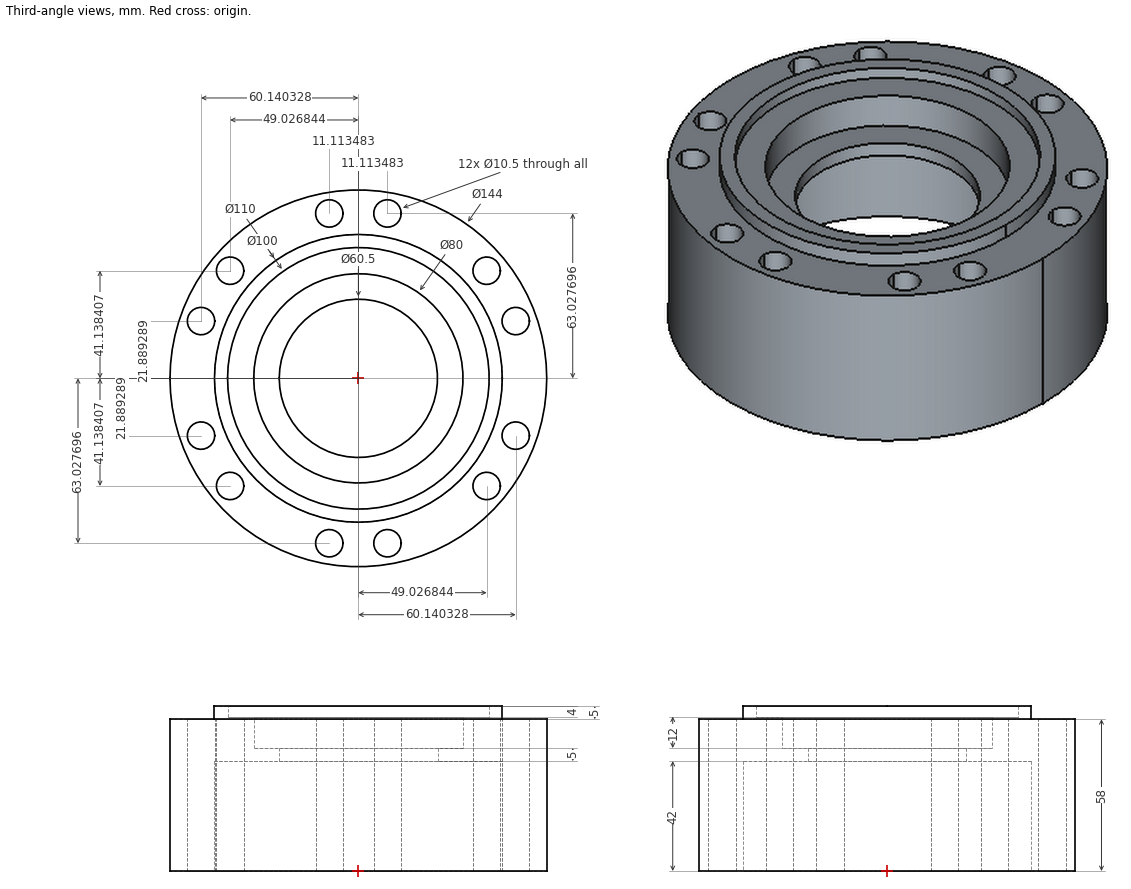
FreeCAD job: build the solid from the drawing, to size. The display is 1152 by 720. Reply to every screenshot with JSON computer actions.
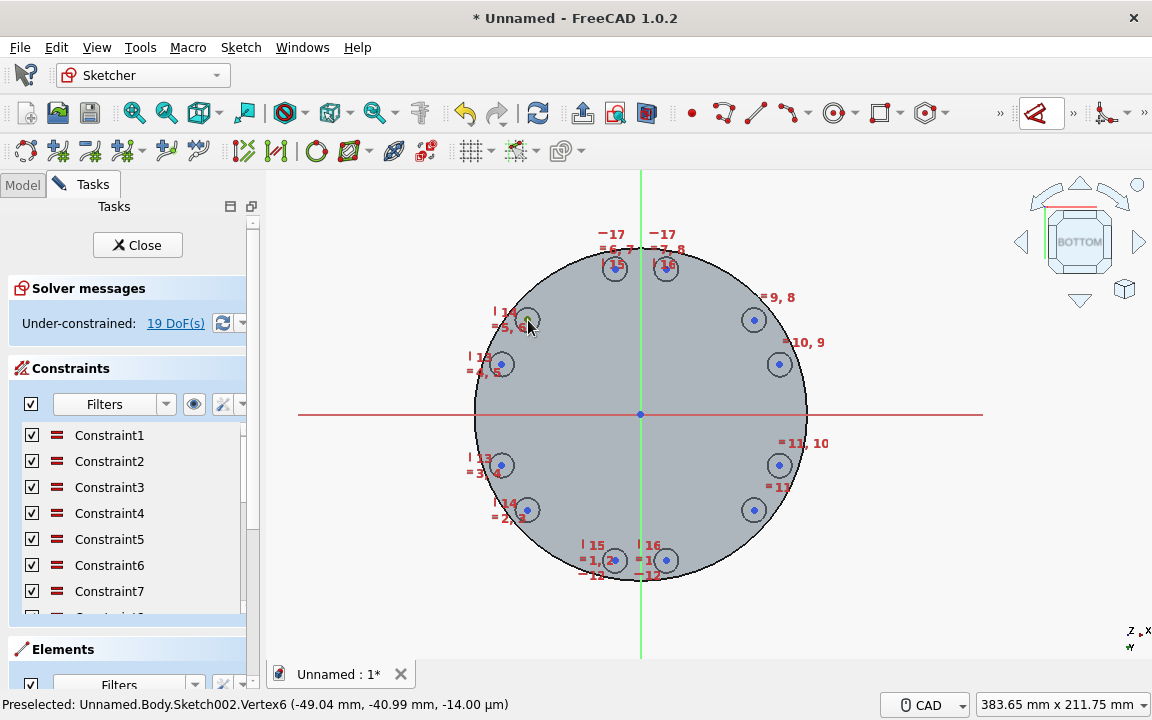
{"action": "left_click", "coordinate": [754, 320]}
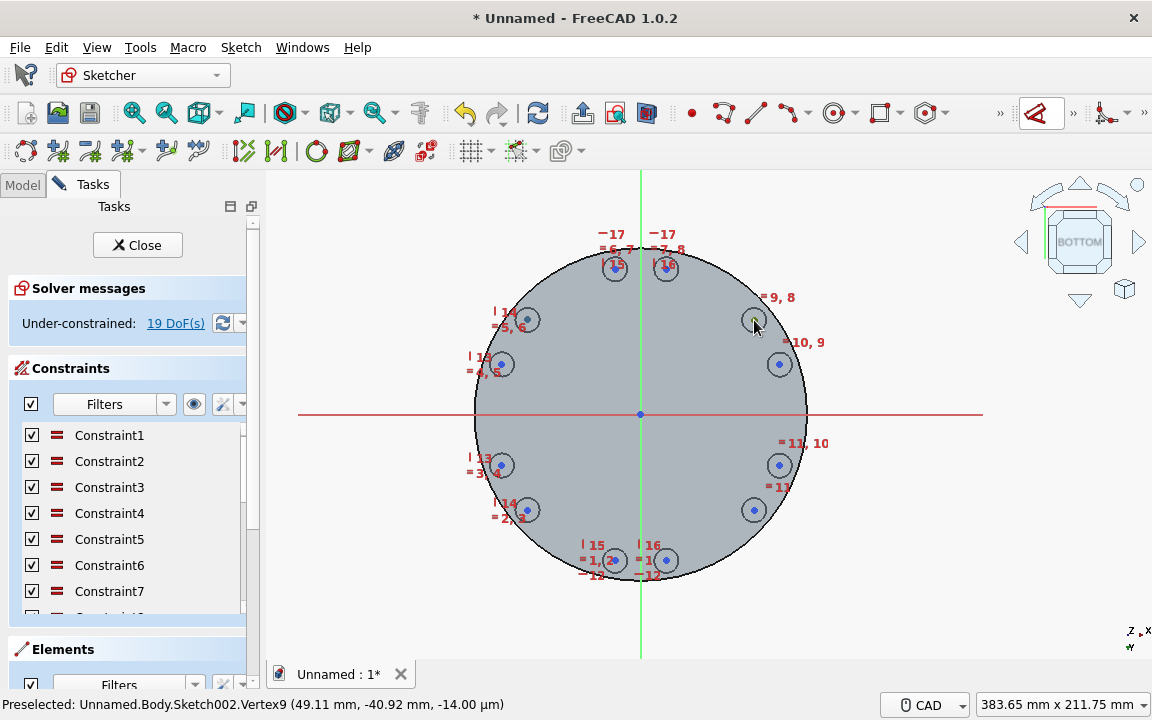
{"action": "key", "text": "h"}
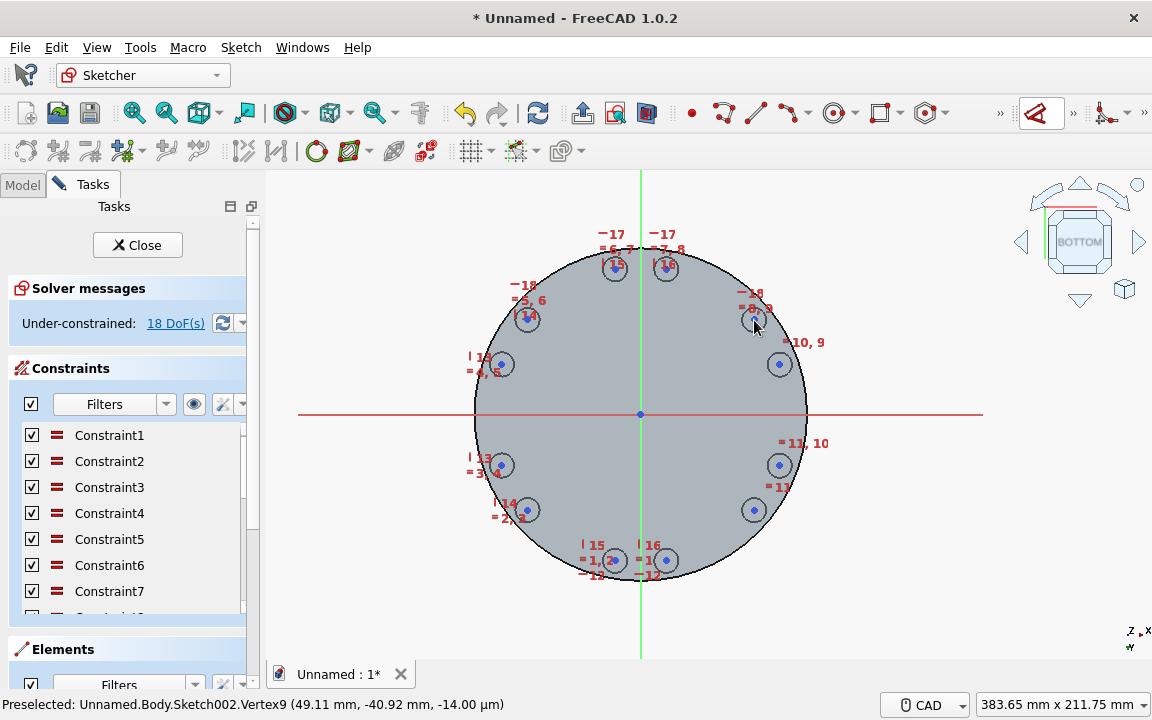
{"action": "left_click", "coordinate": [780, 365]}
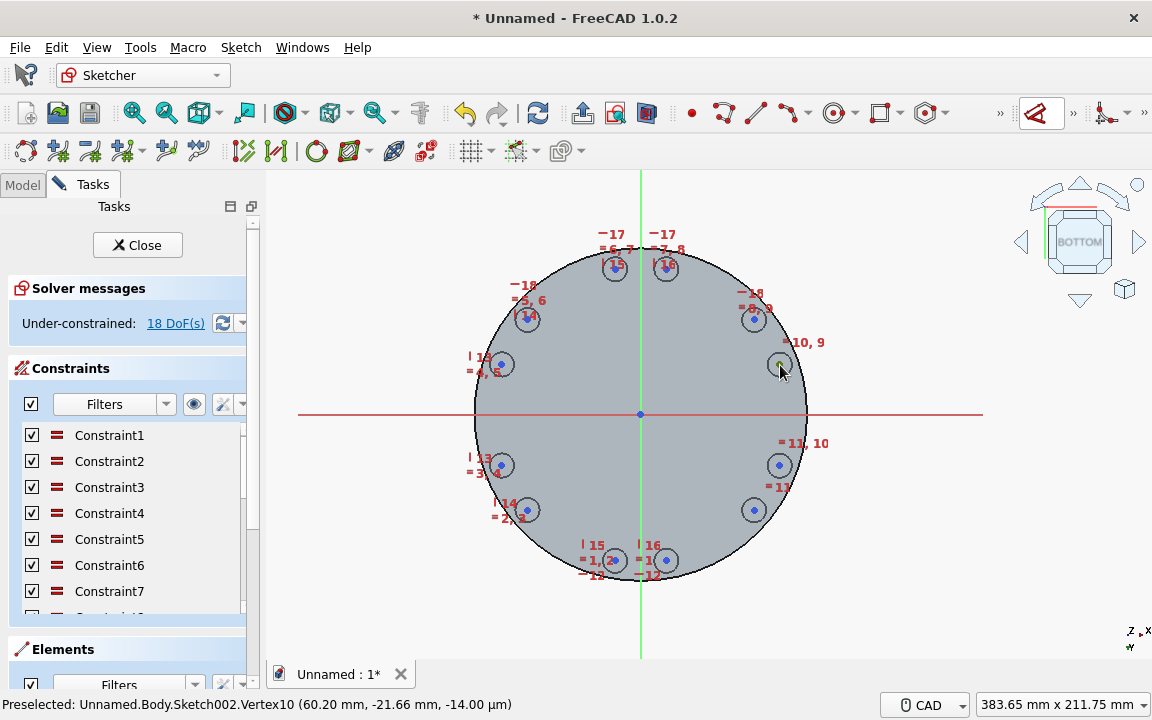
{"action": "left_click", "coordinate": [780, 466]}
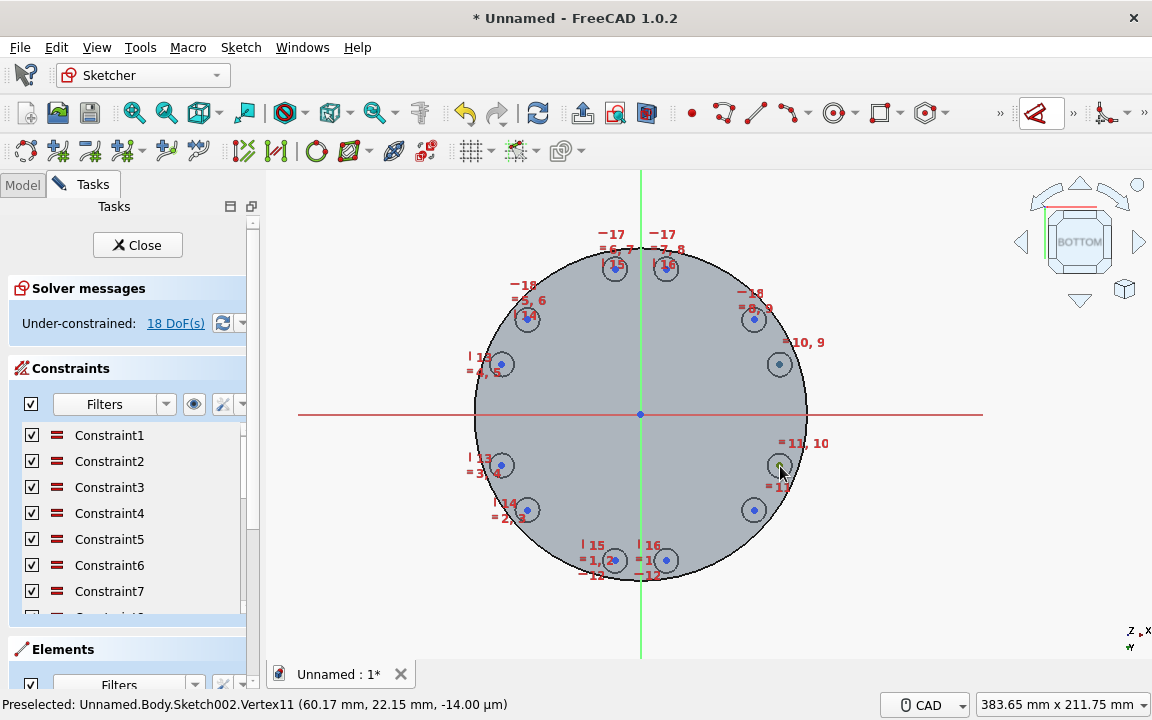
{"action": "key", "text": "v"}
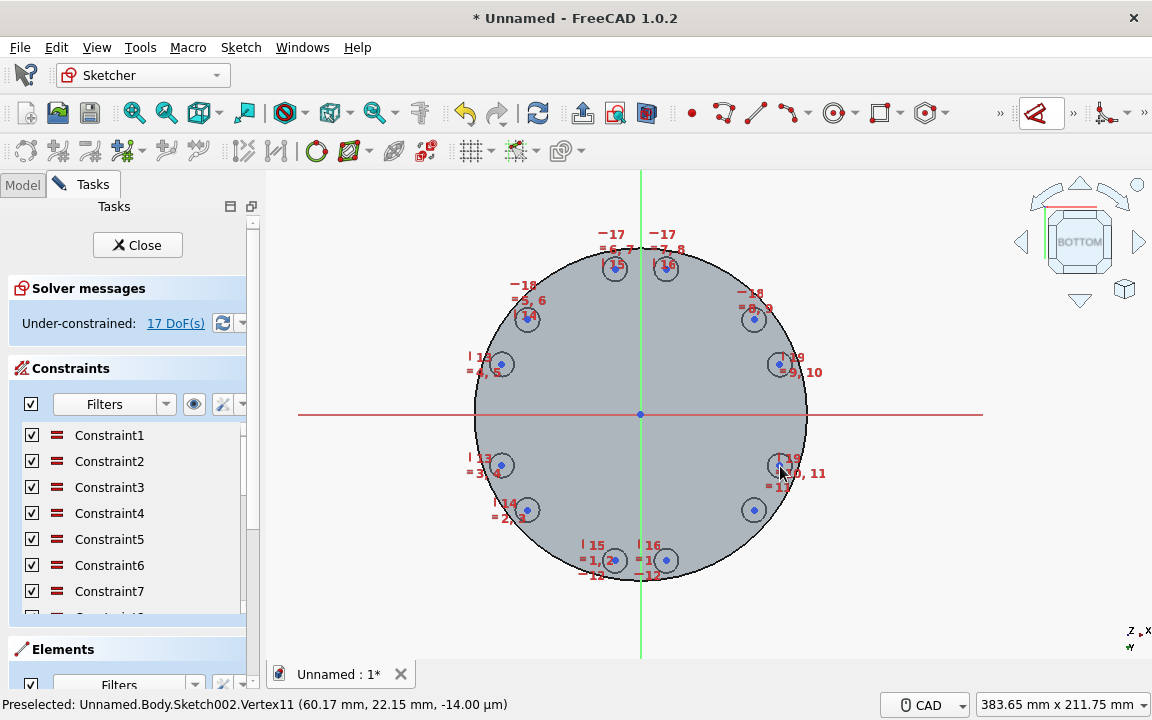
{"action": "left_click", "coordinate": [754, 320]}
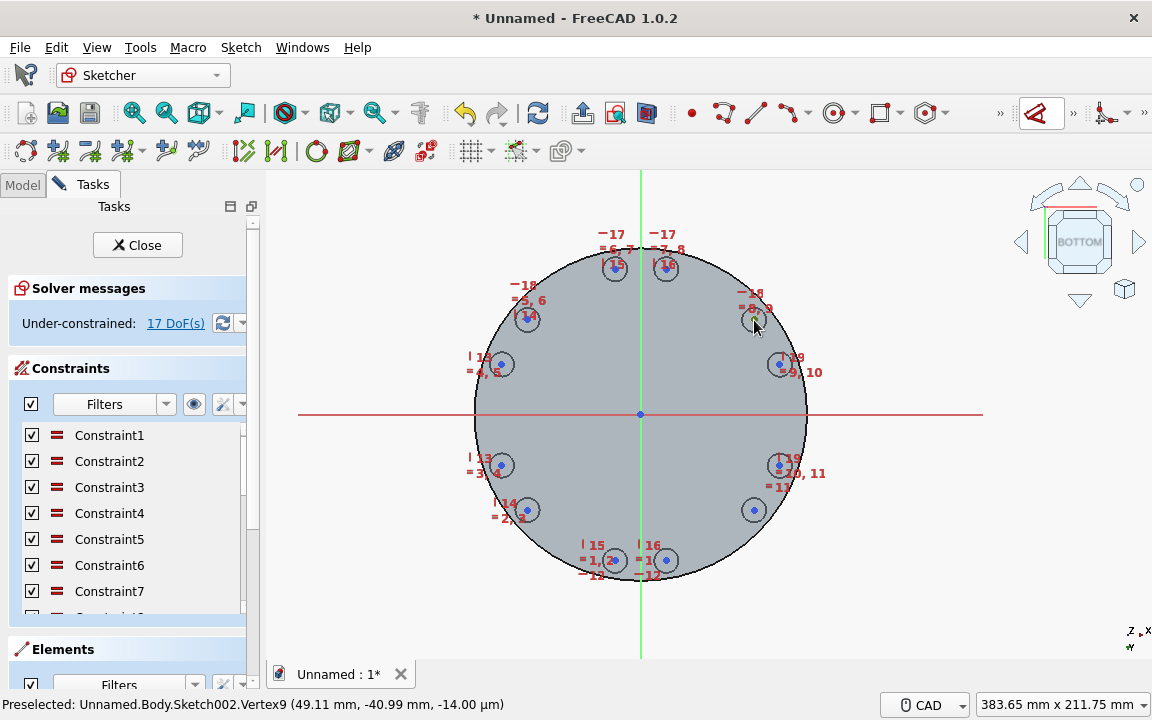
{"action": "left_click", "coordinate": [754, 510]}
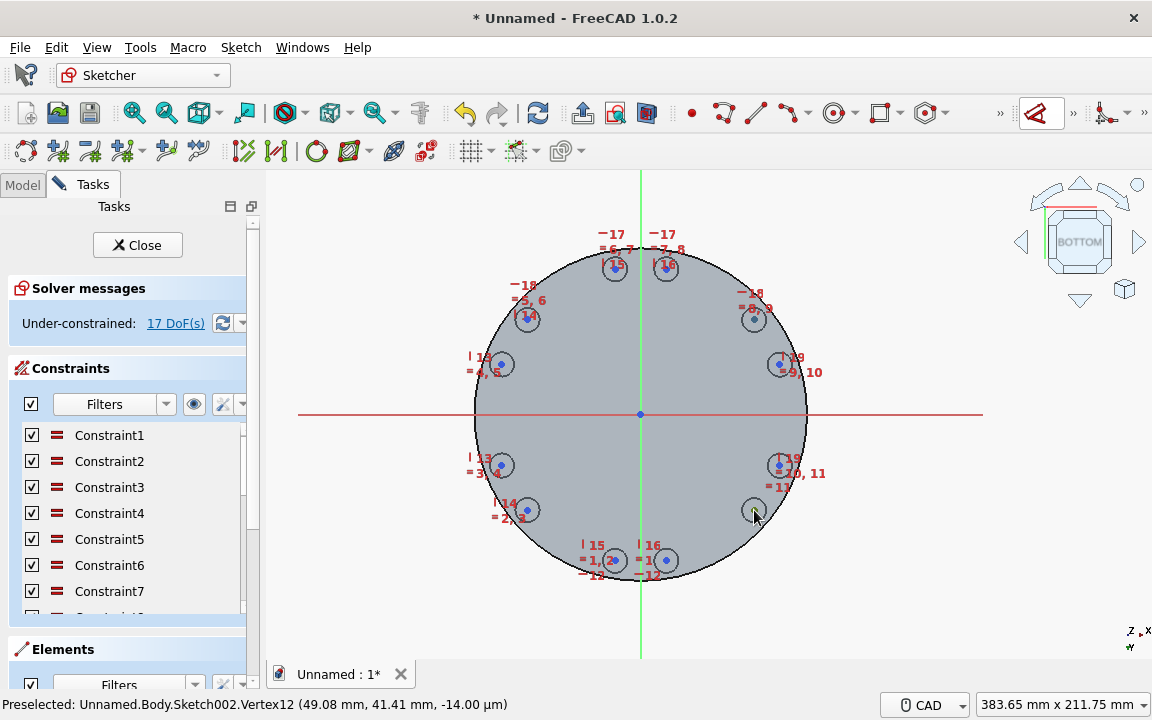
{"action": "key", "text": "v"}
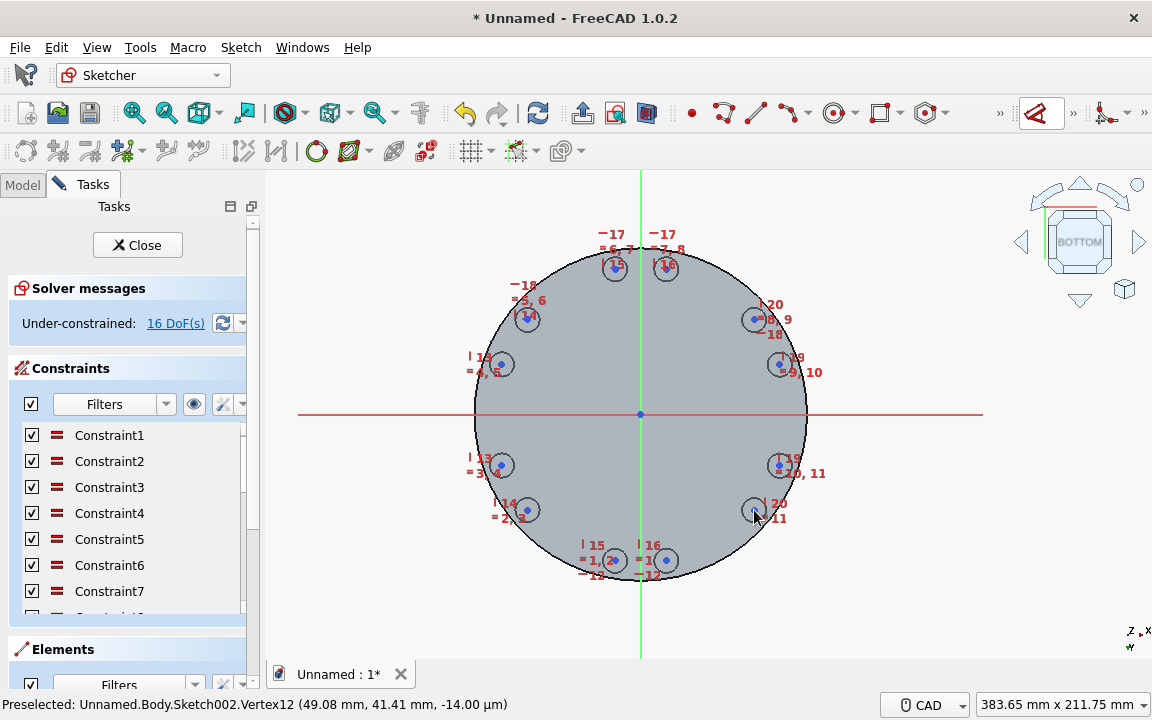
{"action": "left_click", "coordinate": [528, 510]}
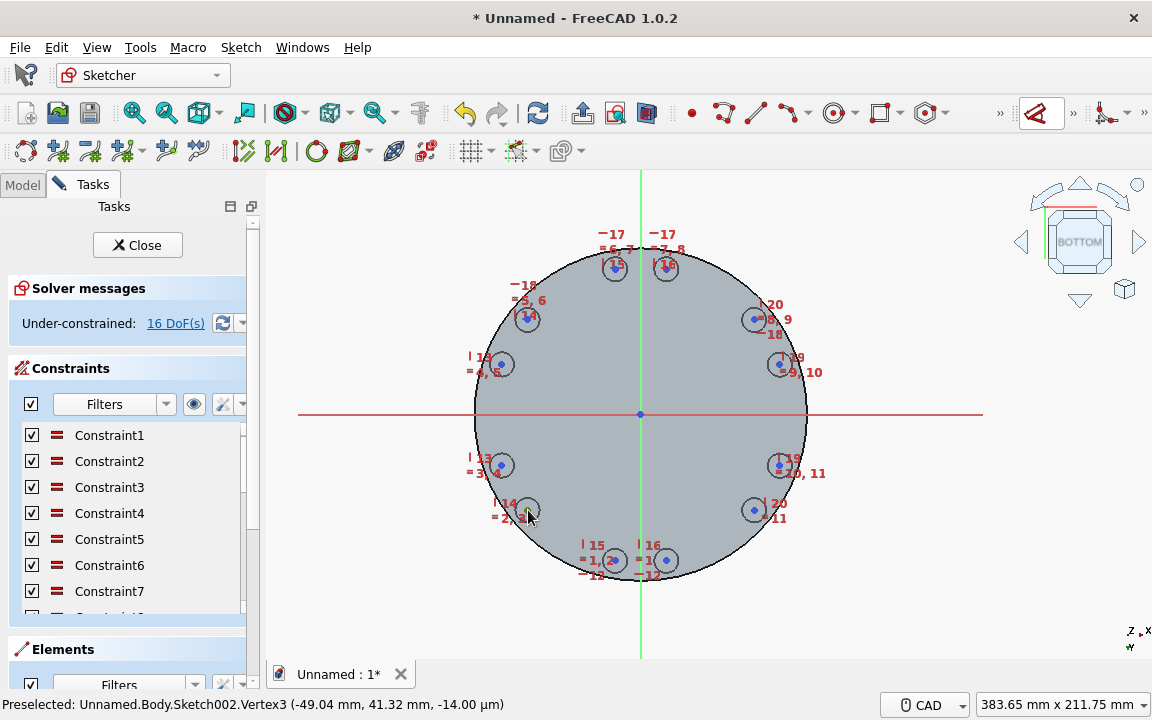
{"action": "left_click", "coordinate": [754, 510]}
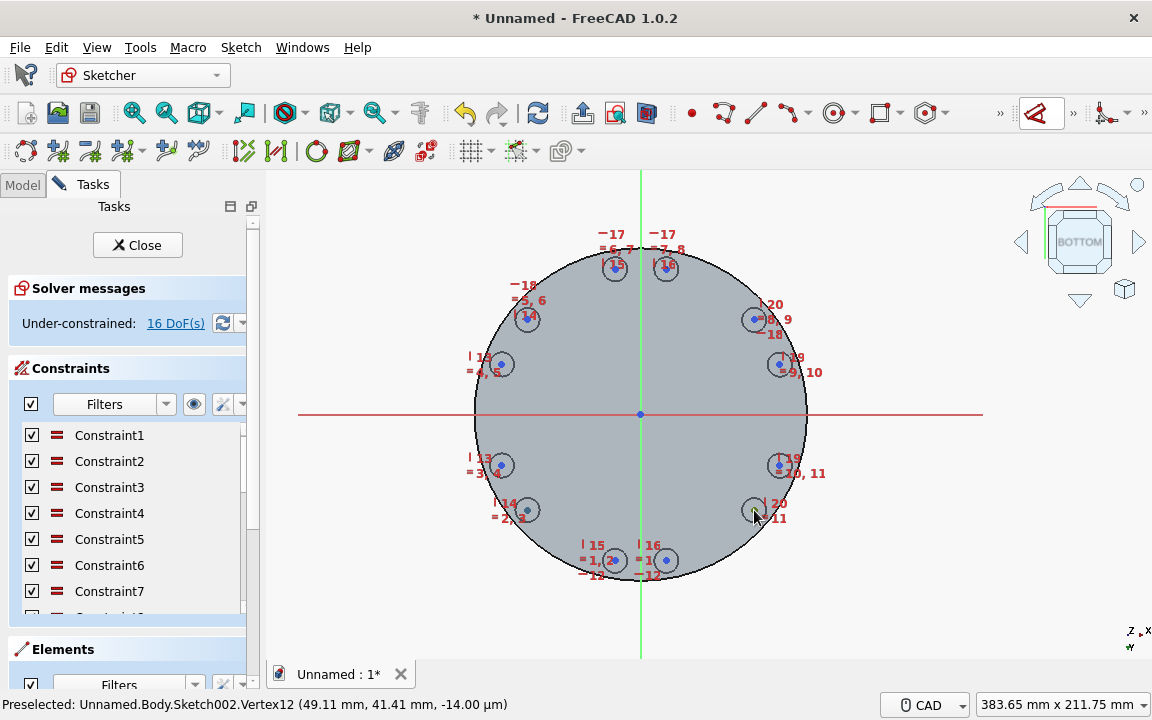
{"action": "key", "text": "h"}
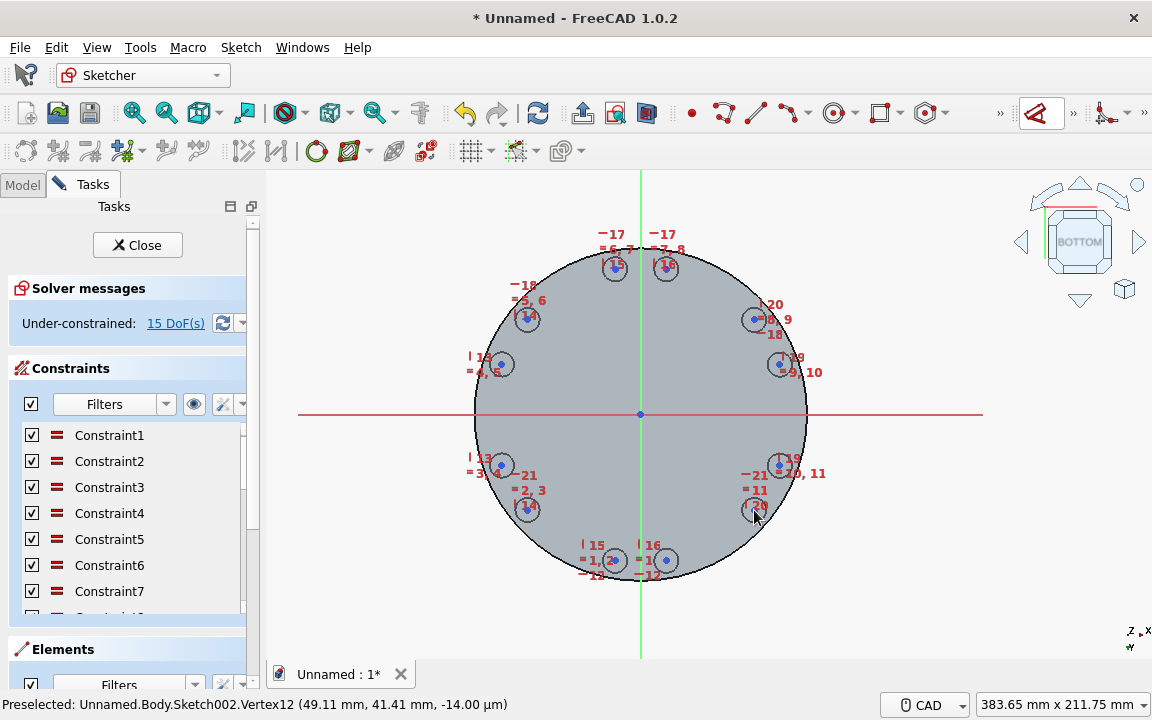
{"action": "key", "text": "d"}